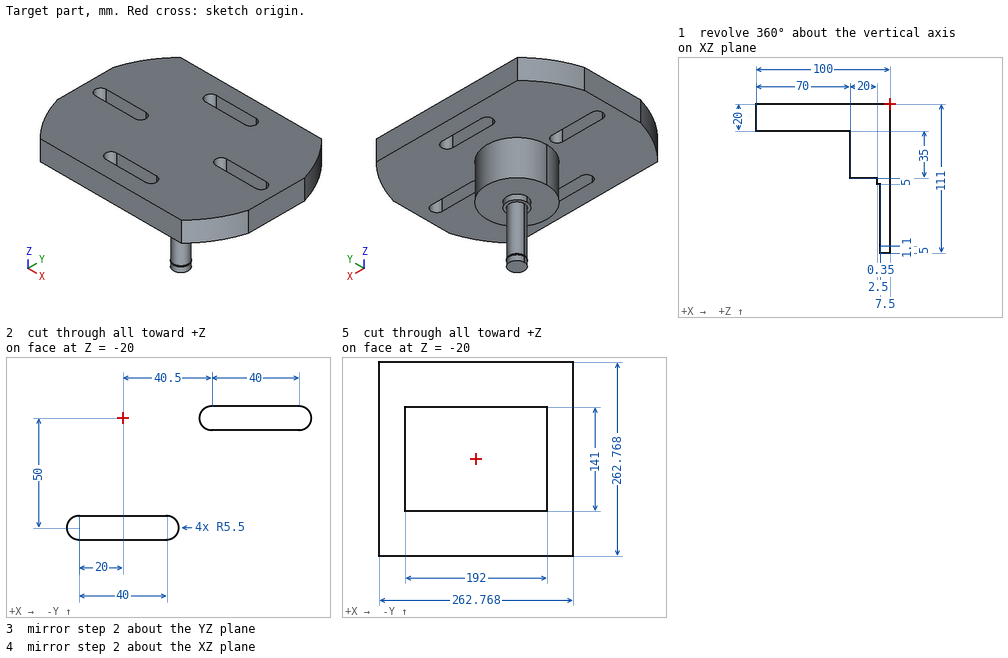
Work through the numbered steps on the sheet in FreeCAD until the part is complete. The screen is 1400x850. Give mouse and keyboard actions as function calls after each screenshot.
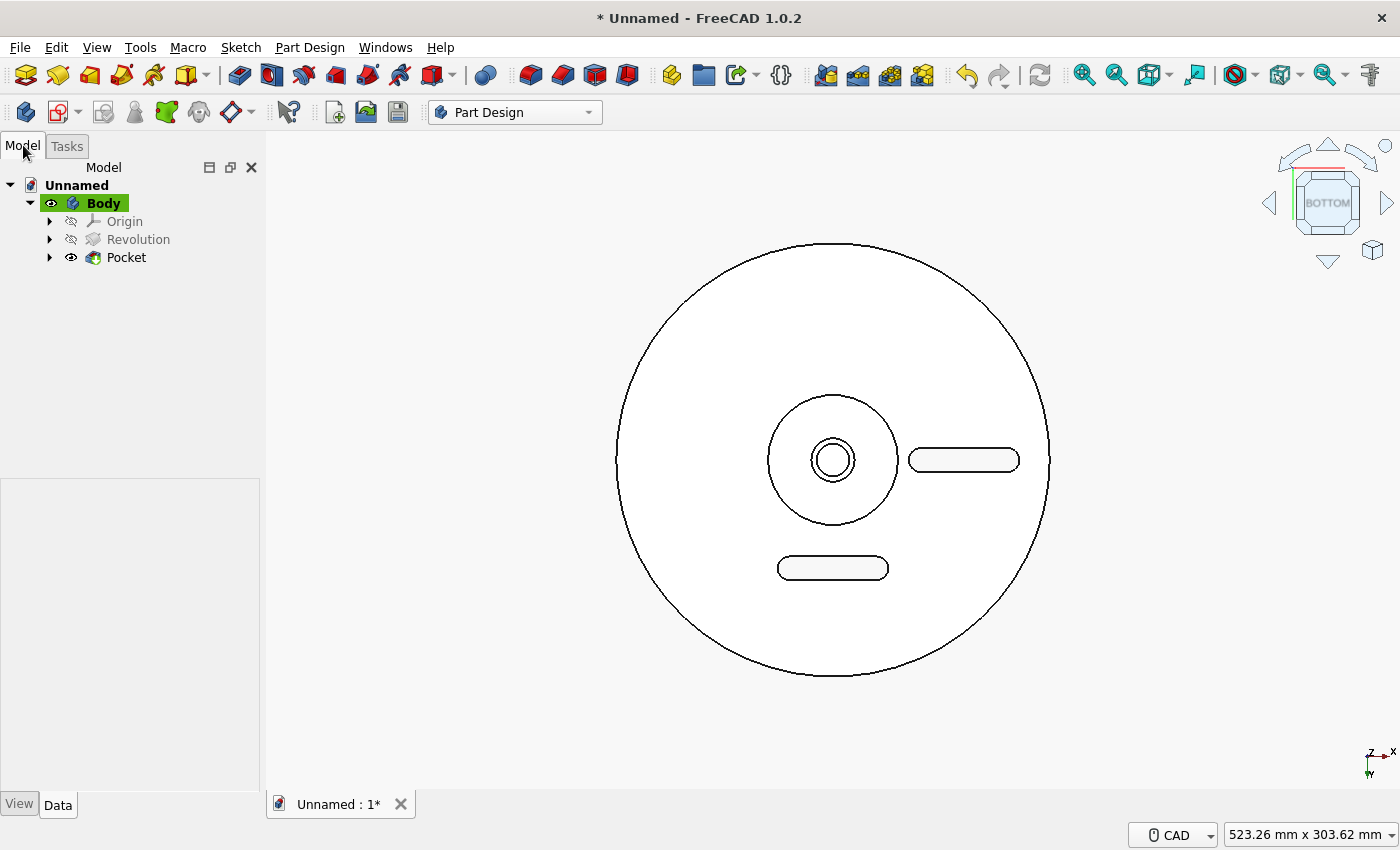
click(116, 257)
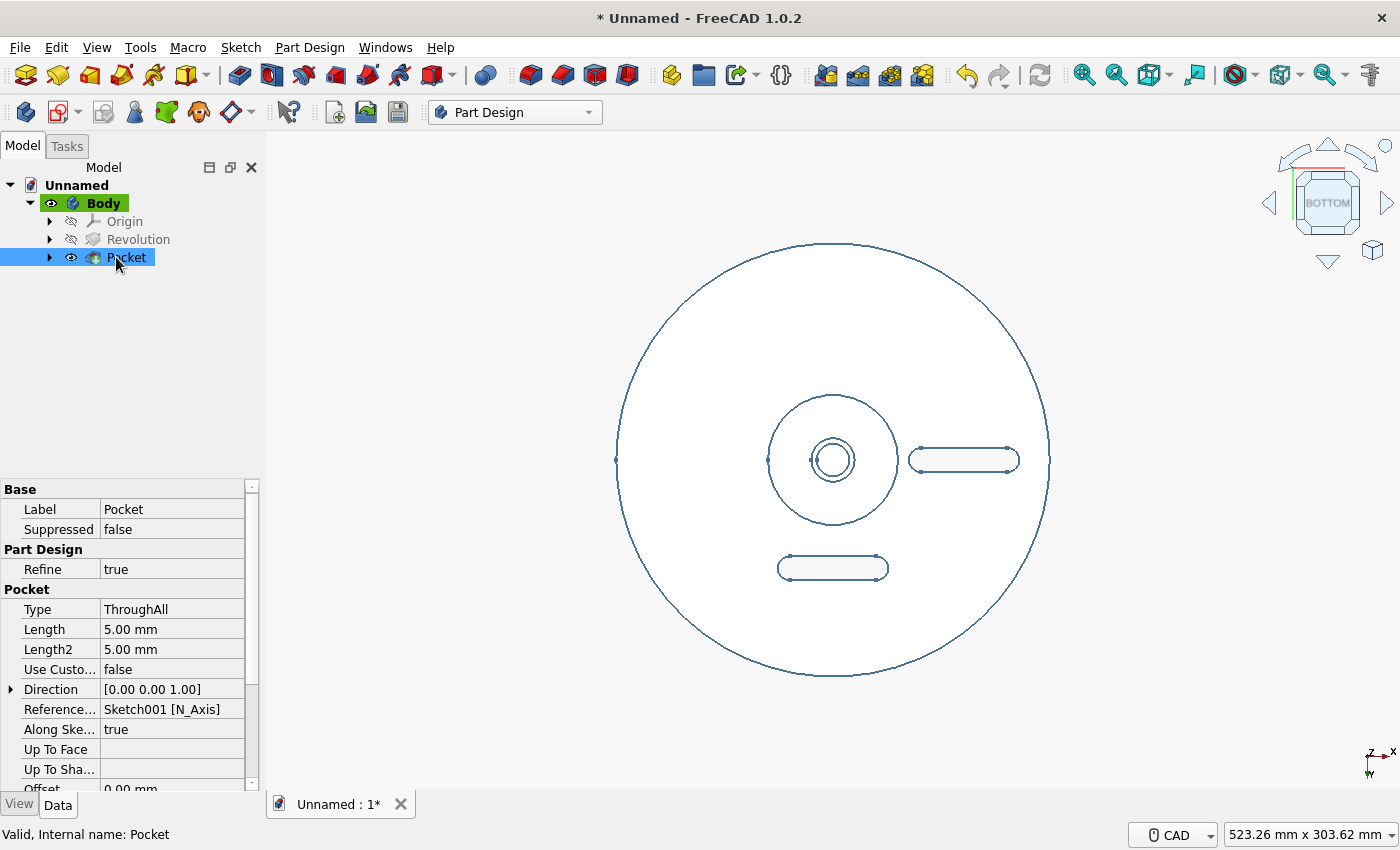
click(826, 76)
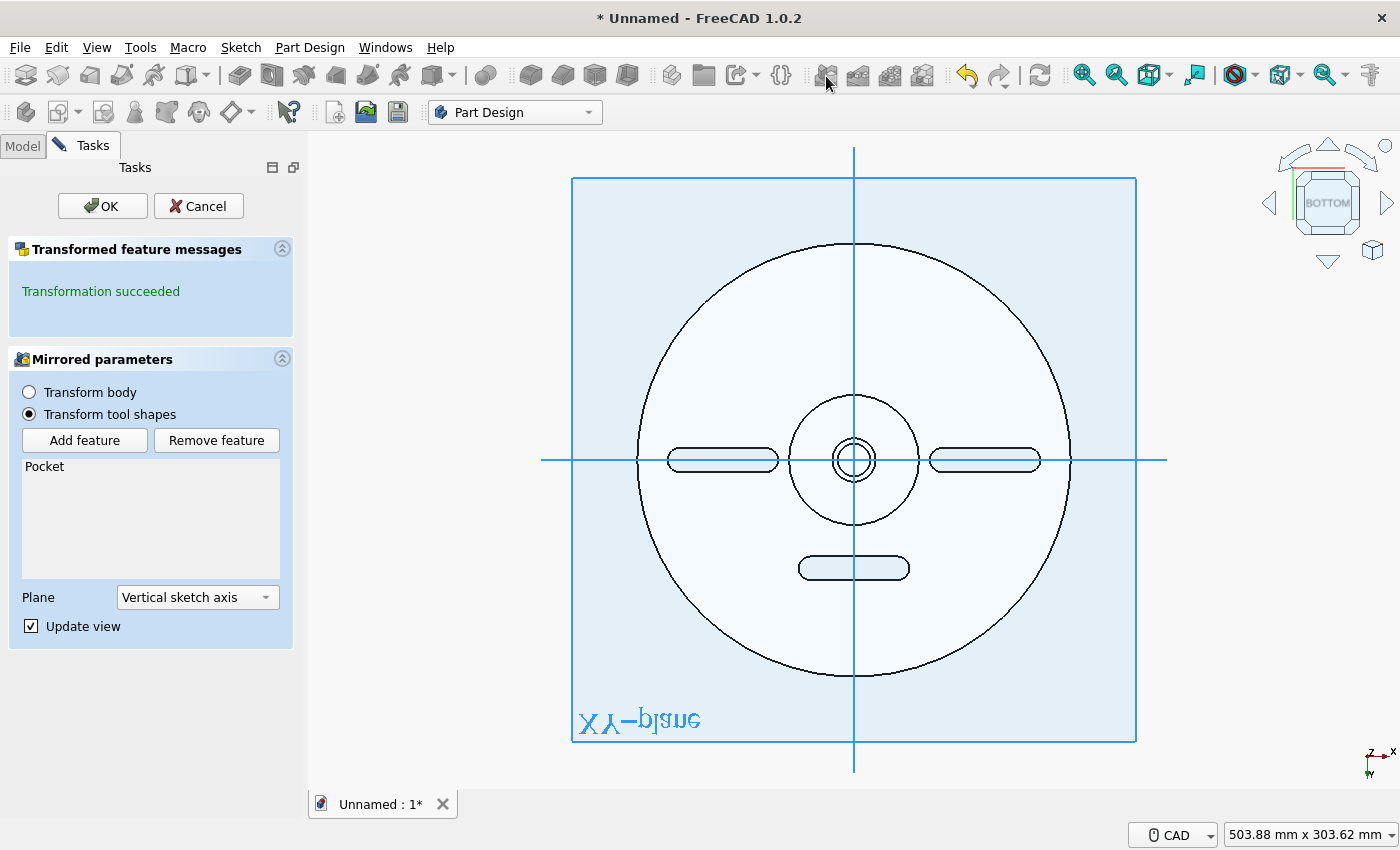
click(198, 598)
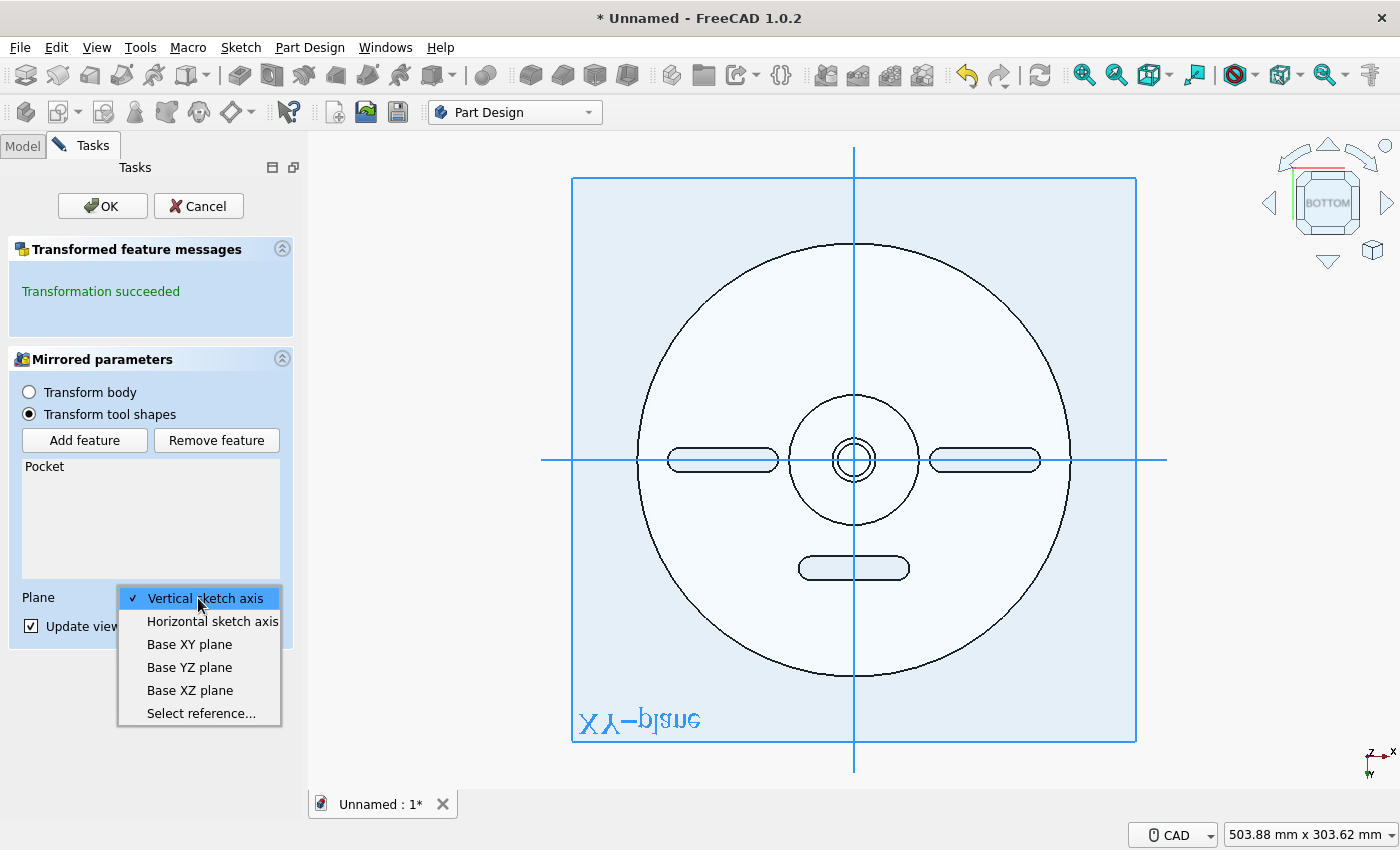
click(198, 668)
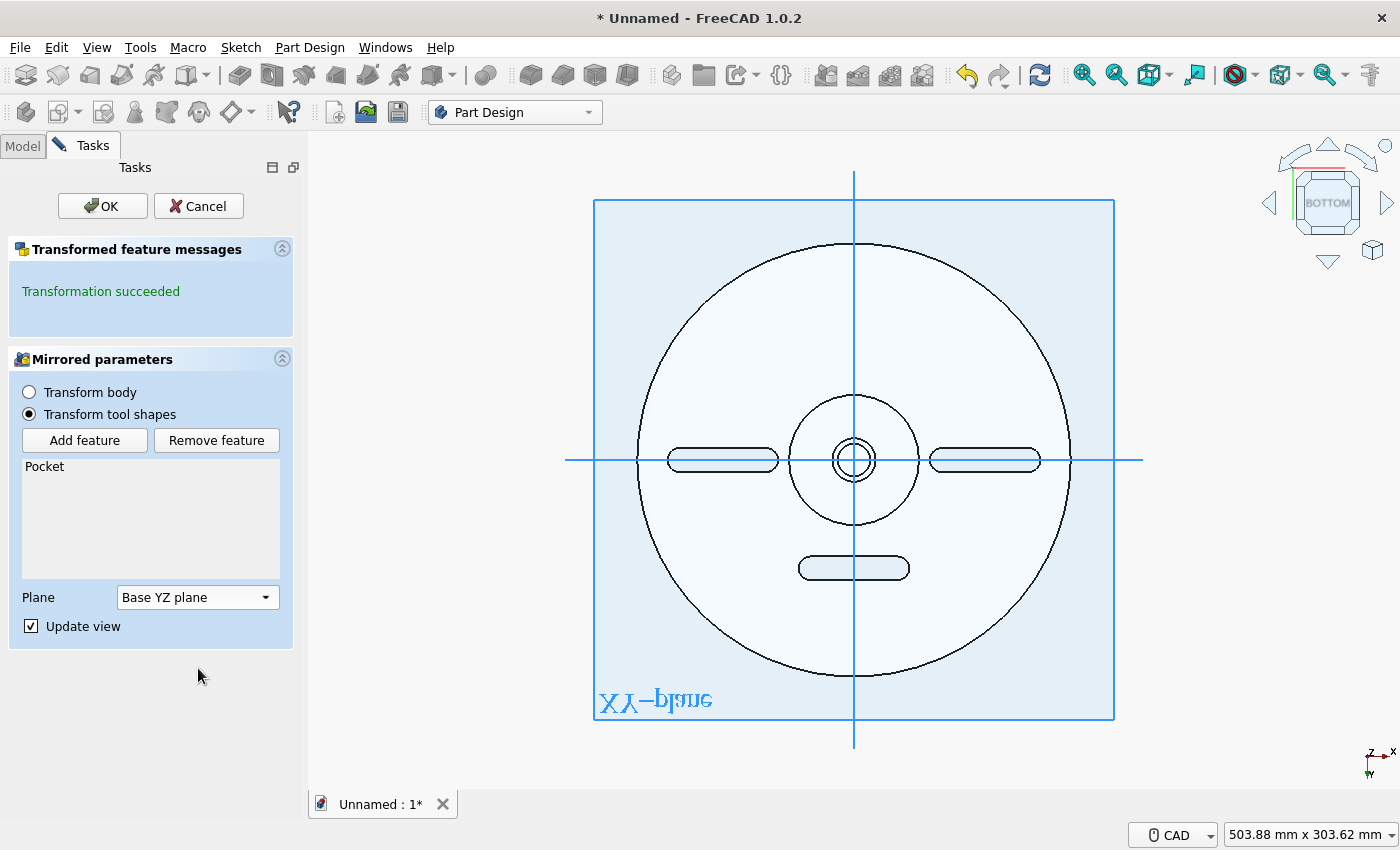
click(103, 206)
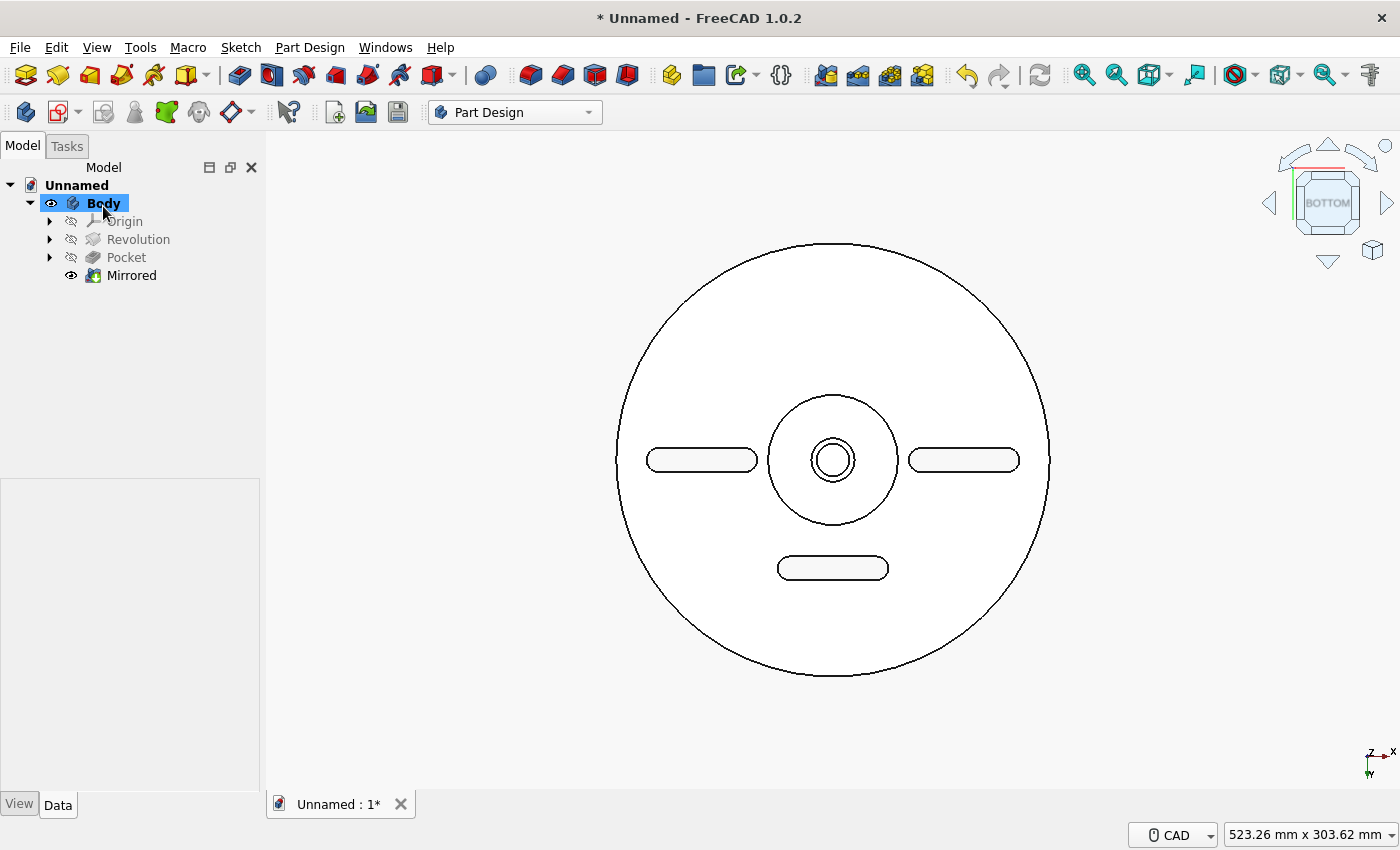
click(116, 257)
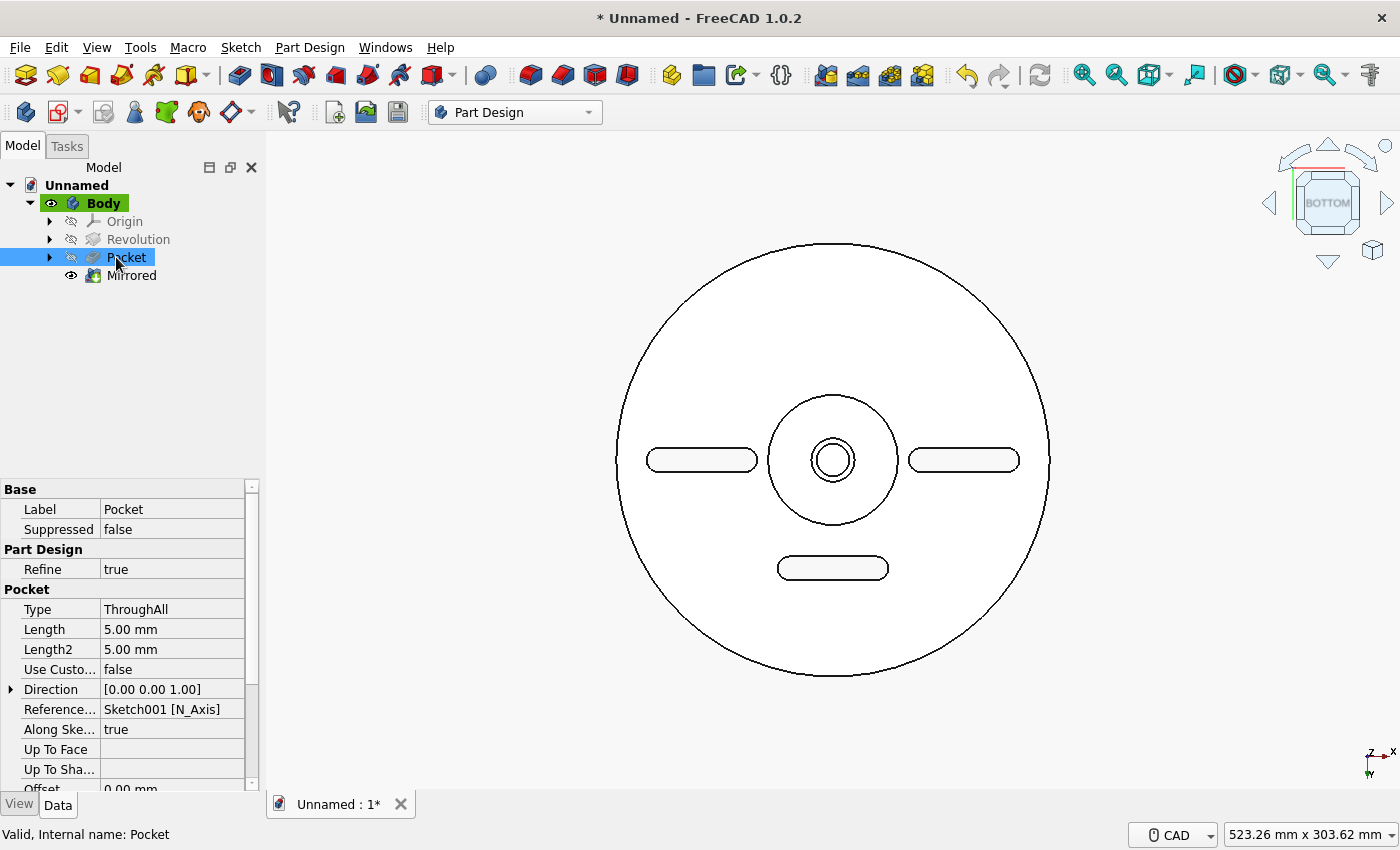
click(826, 76)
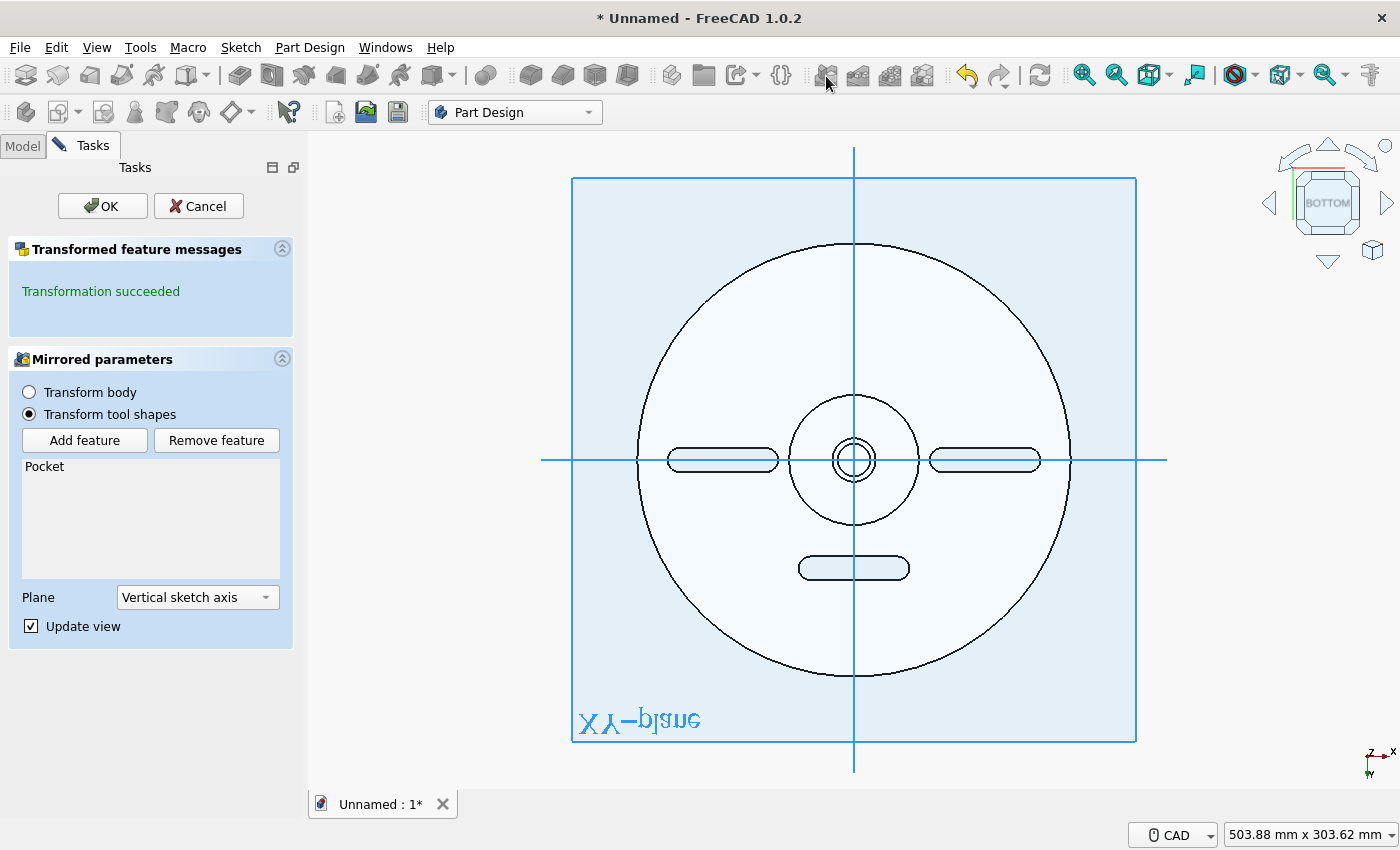
click(198, 598)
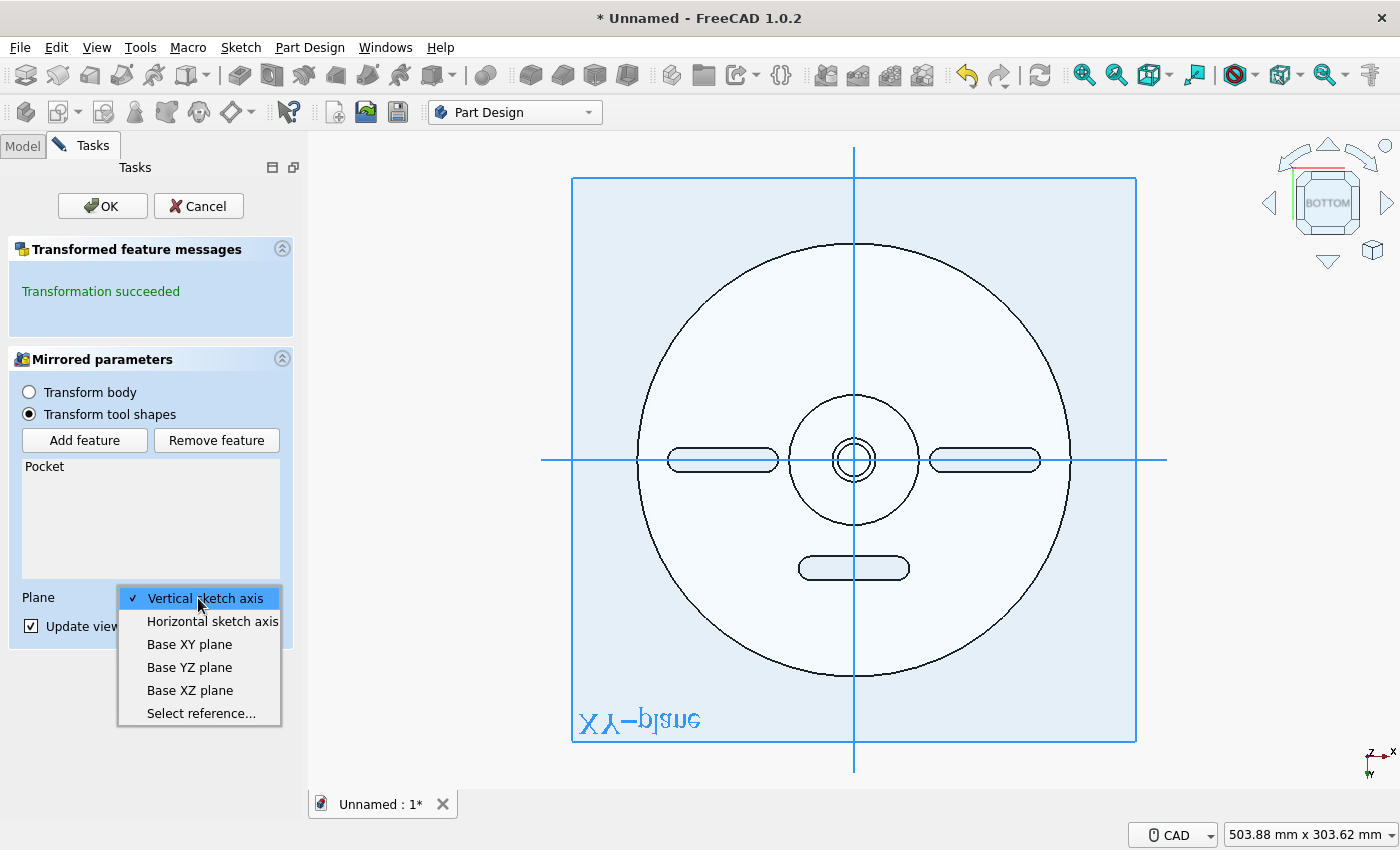
click(198, 690)